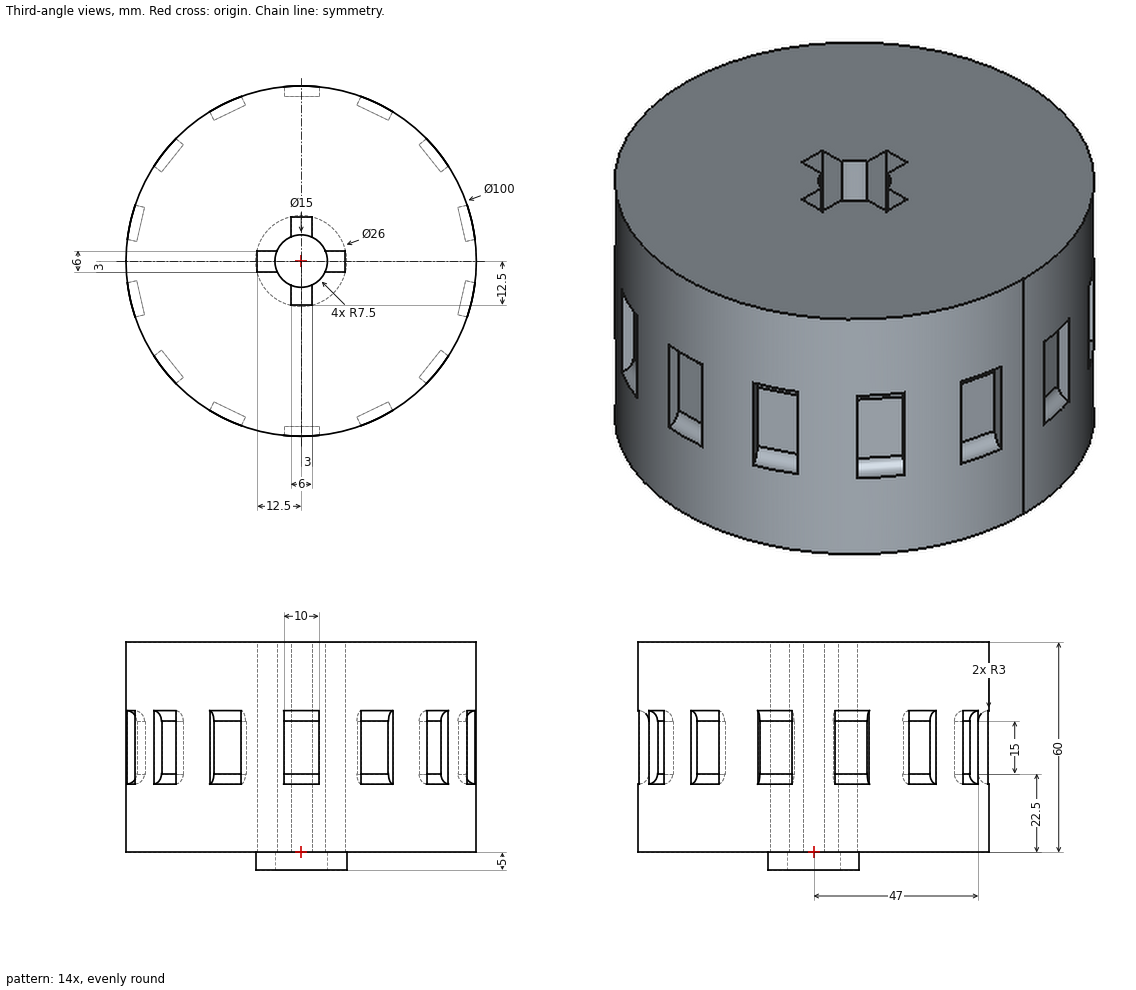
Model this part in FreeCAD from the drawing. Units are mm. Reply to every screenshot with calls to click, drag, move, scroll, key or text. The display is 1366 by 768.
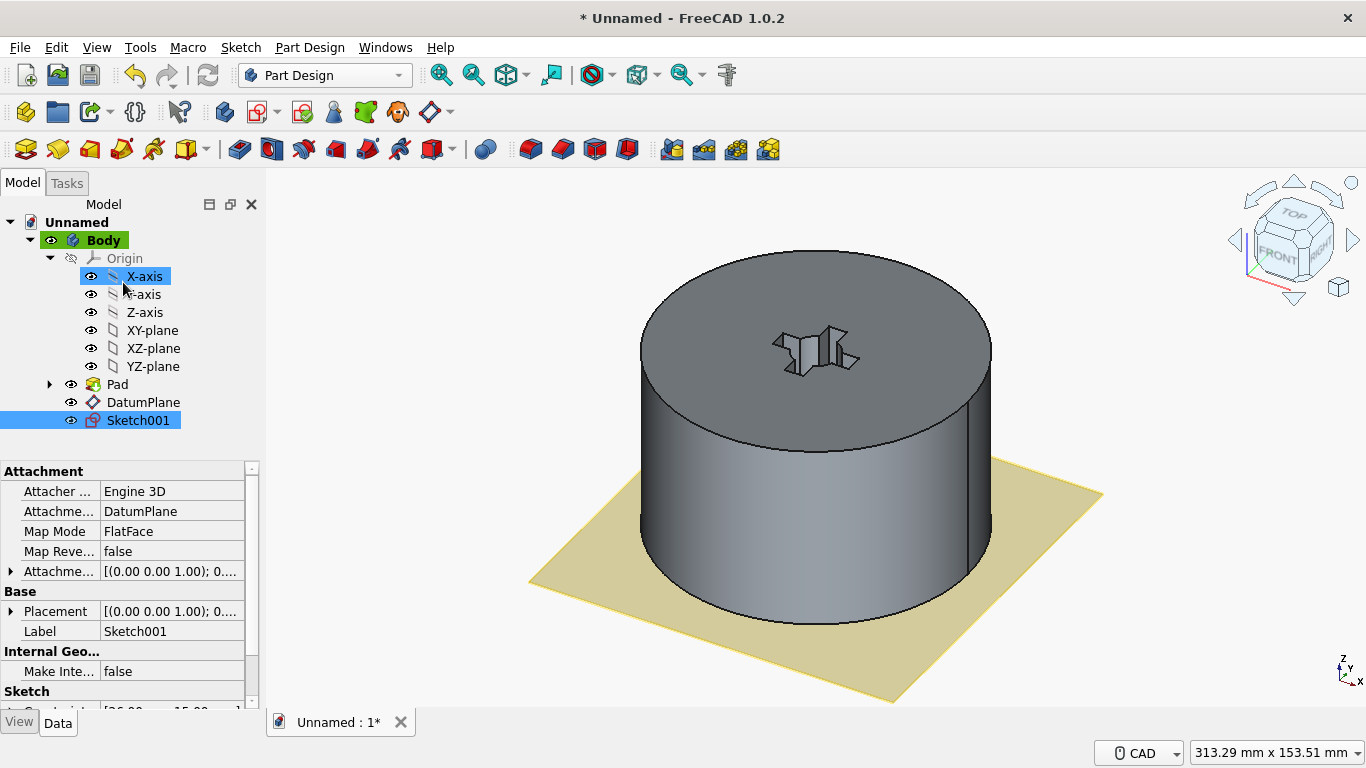
click(26, 150)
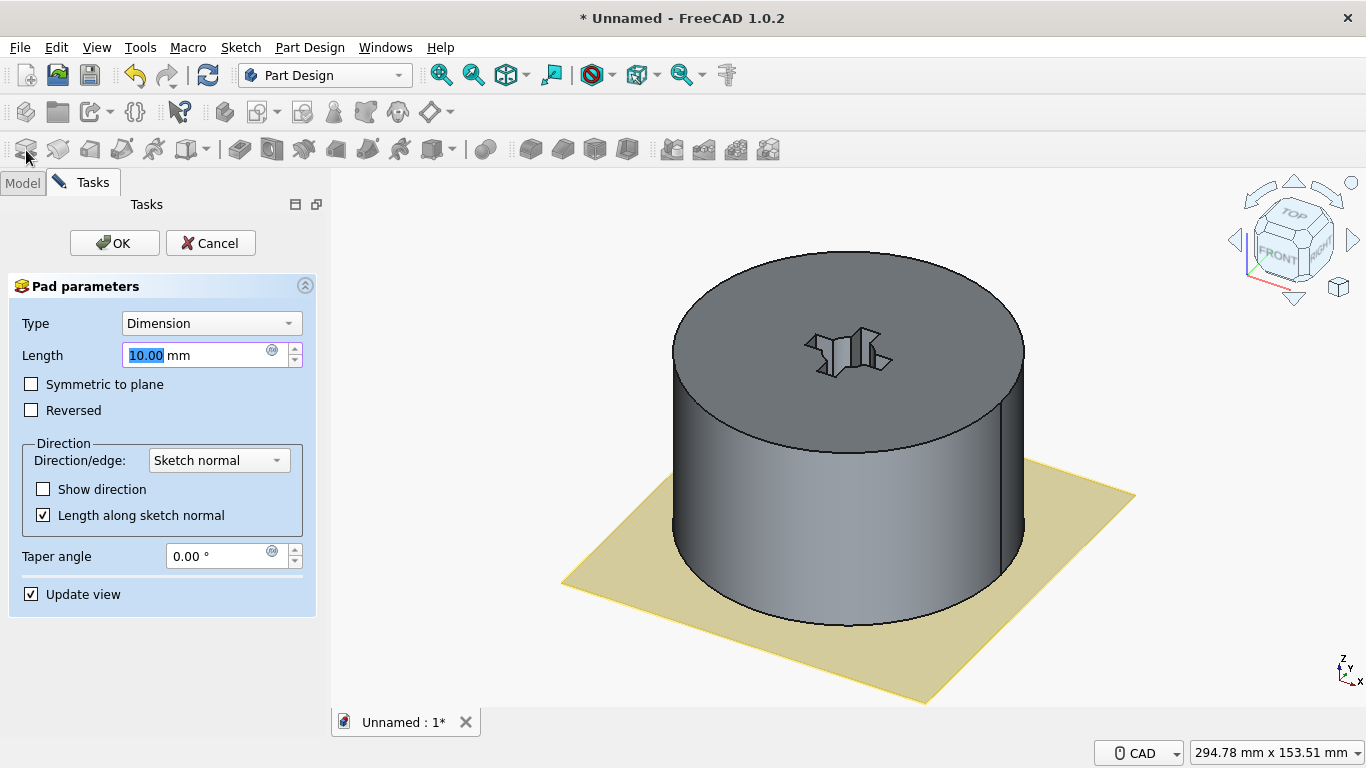
text(5)
key(Tab)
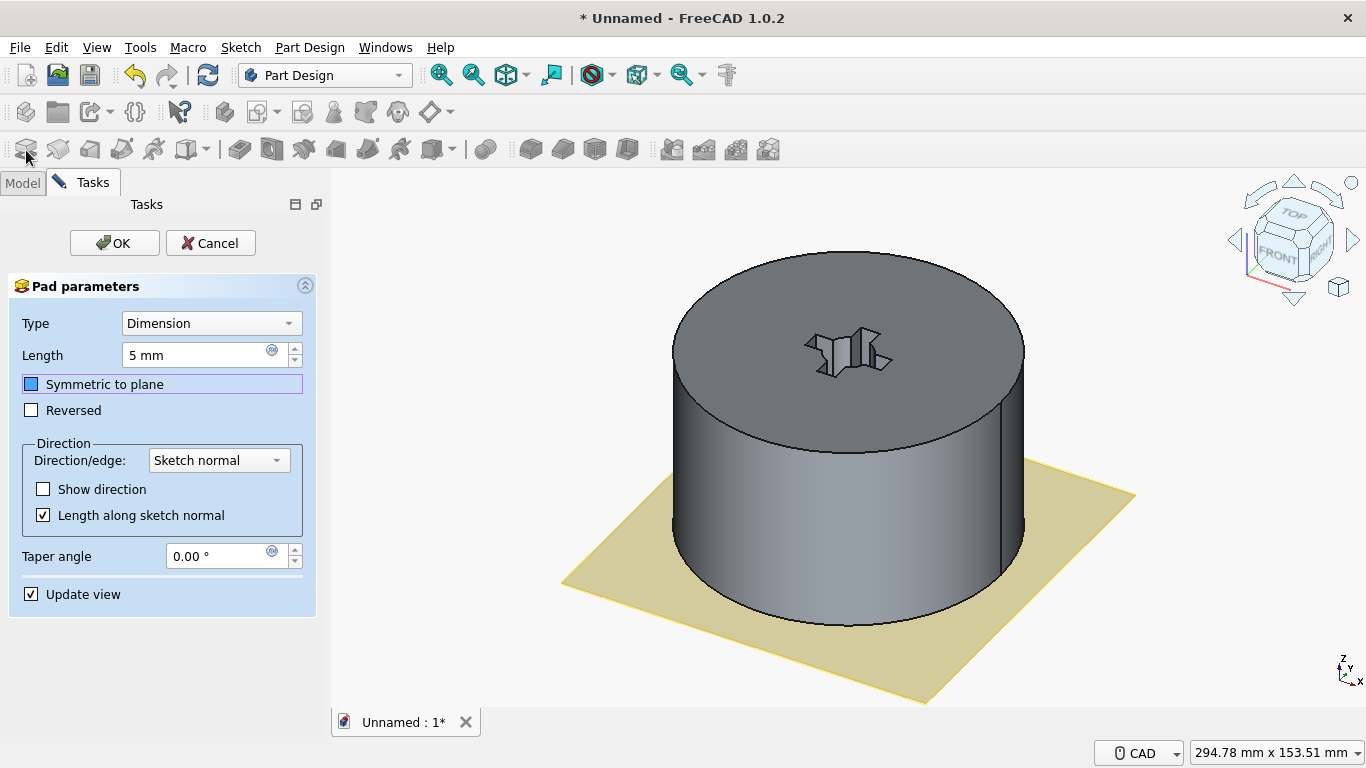
click(115, 243)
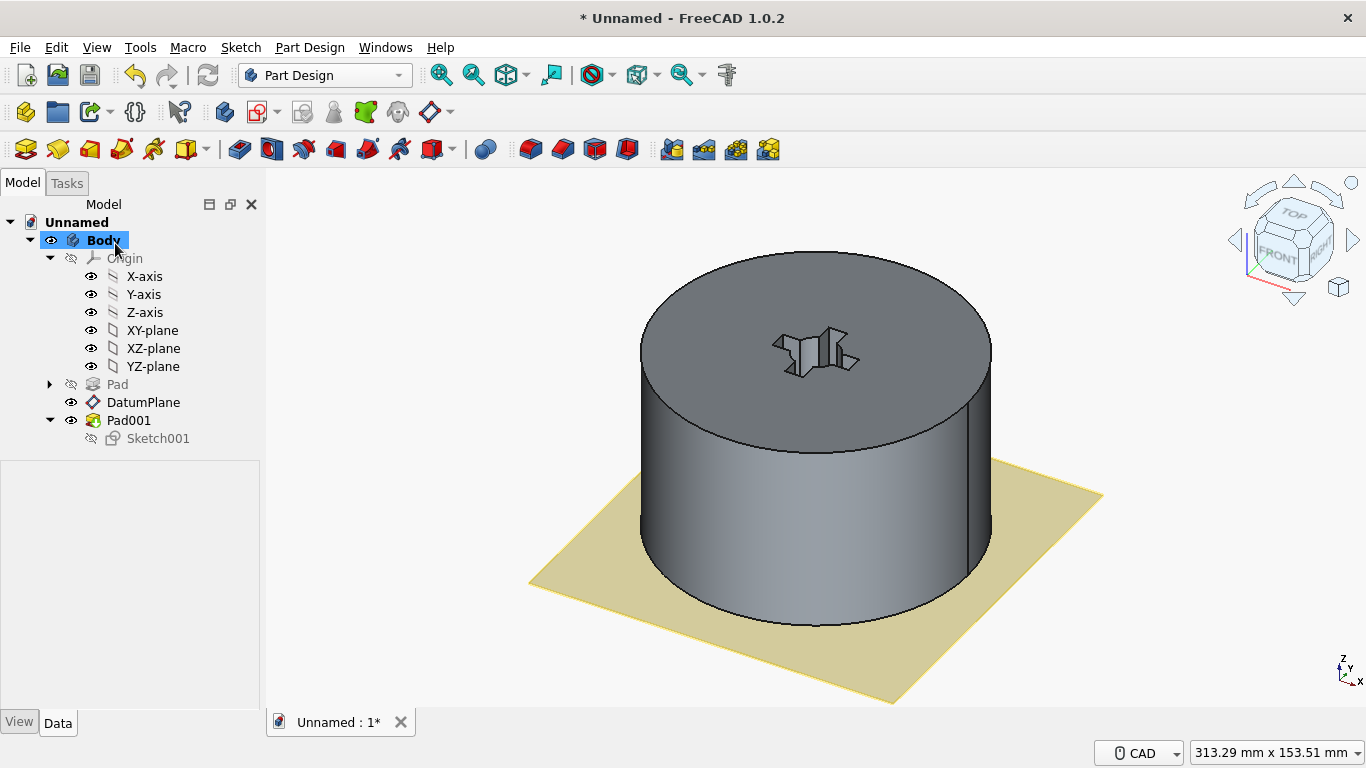
click(116, 402)
key(space)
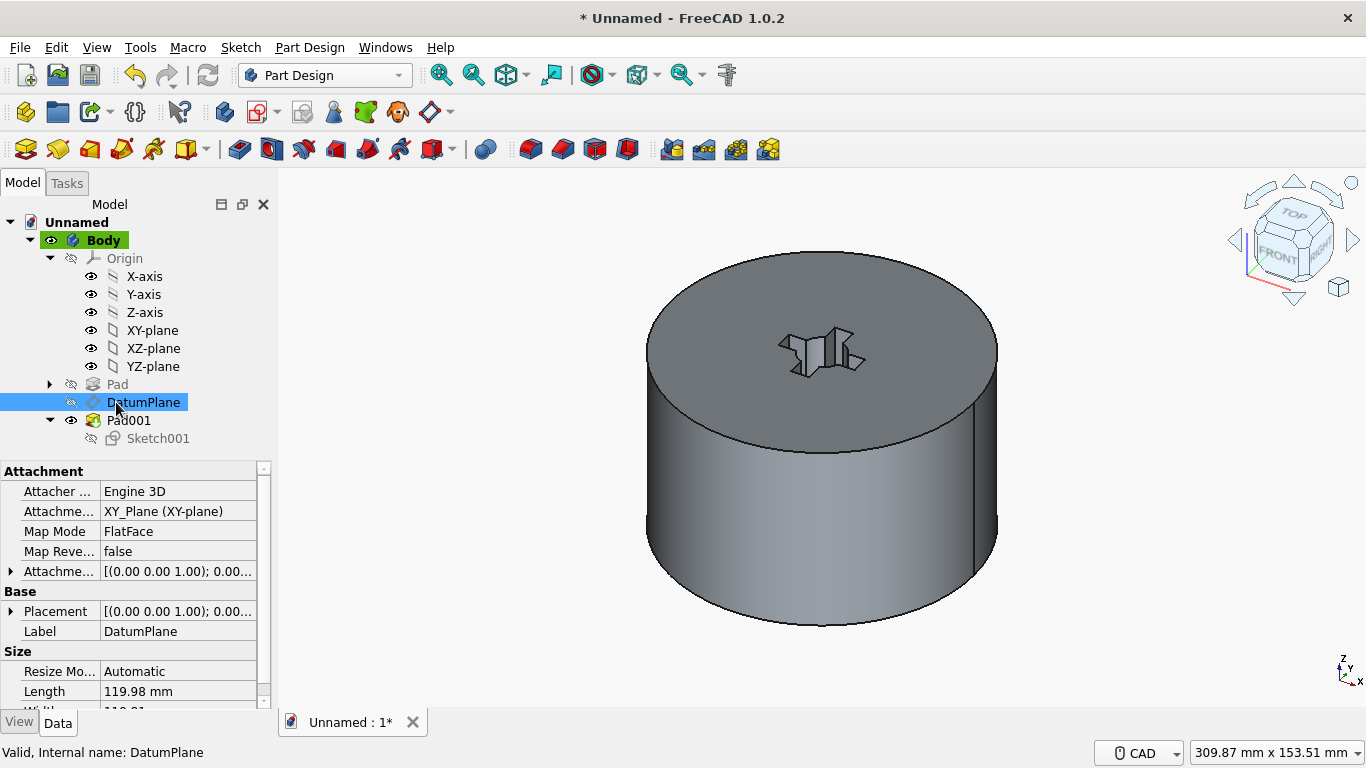
click(318, 667)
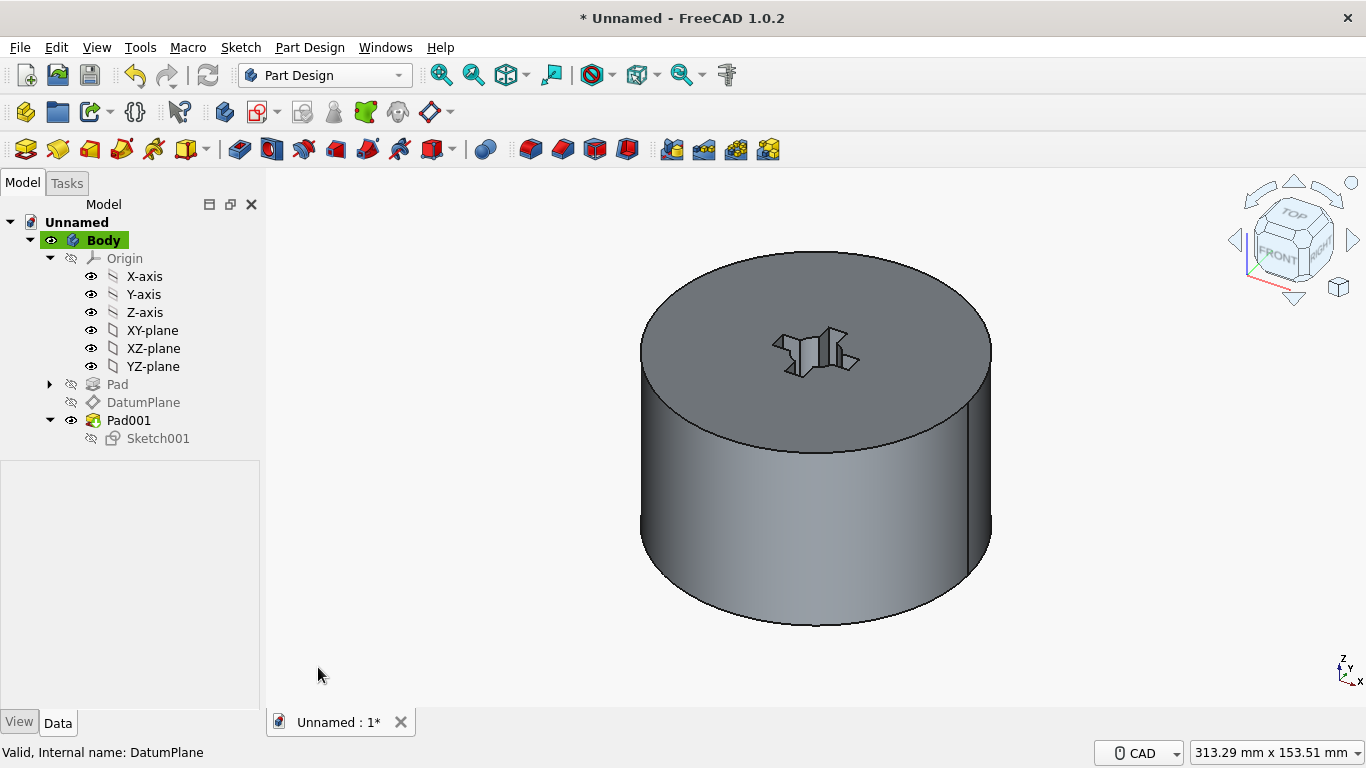
click(258, 112)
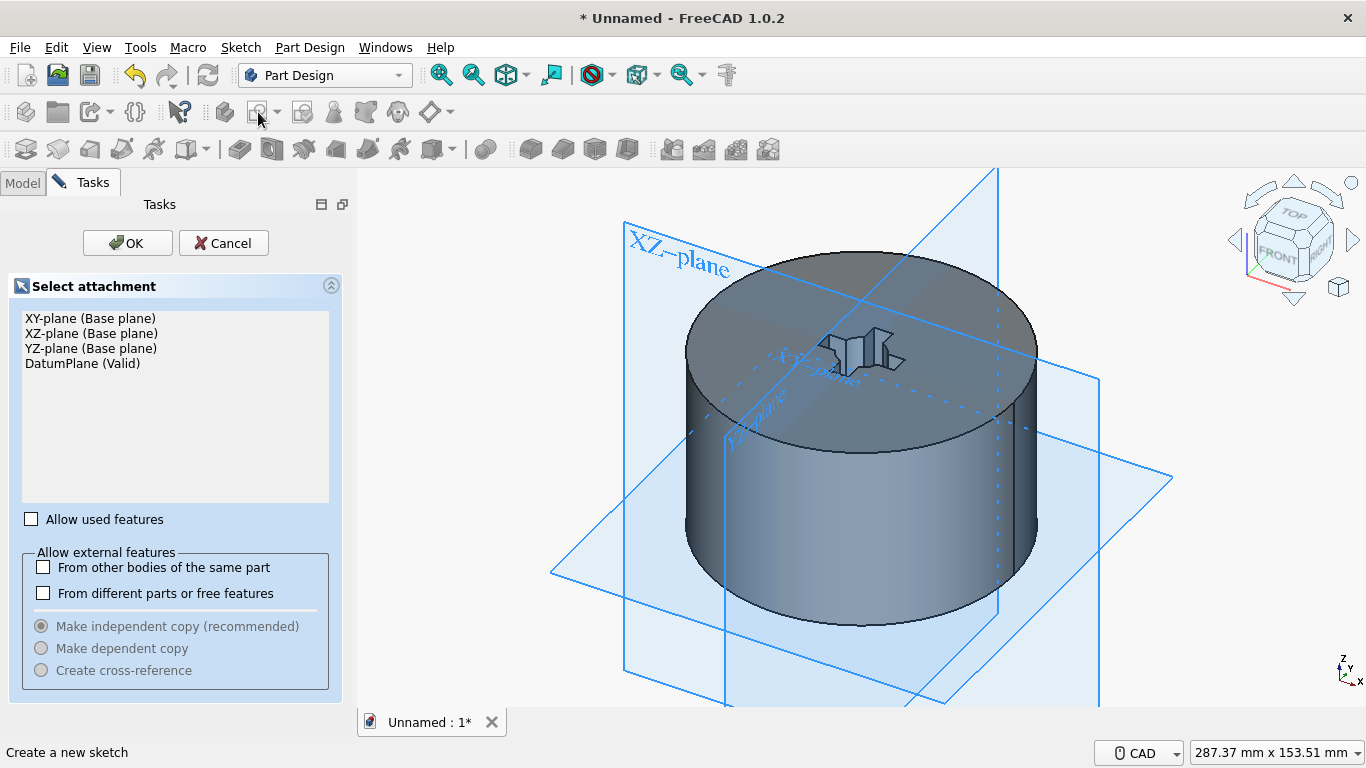
click(82, 348)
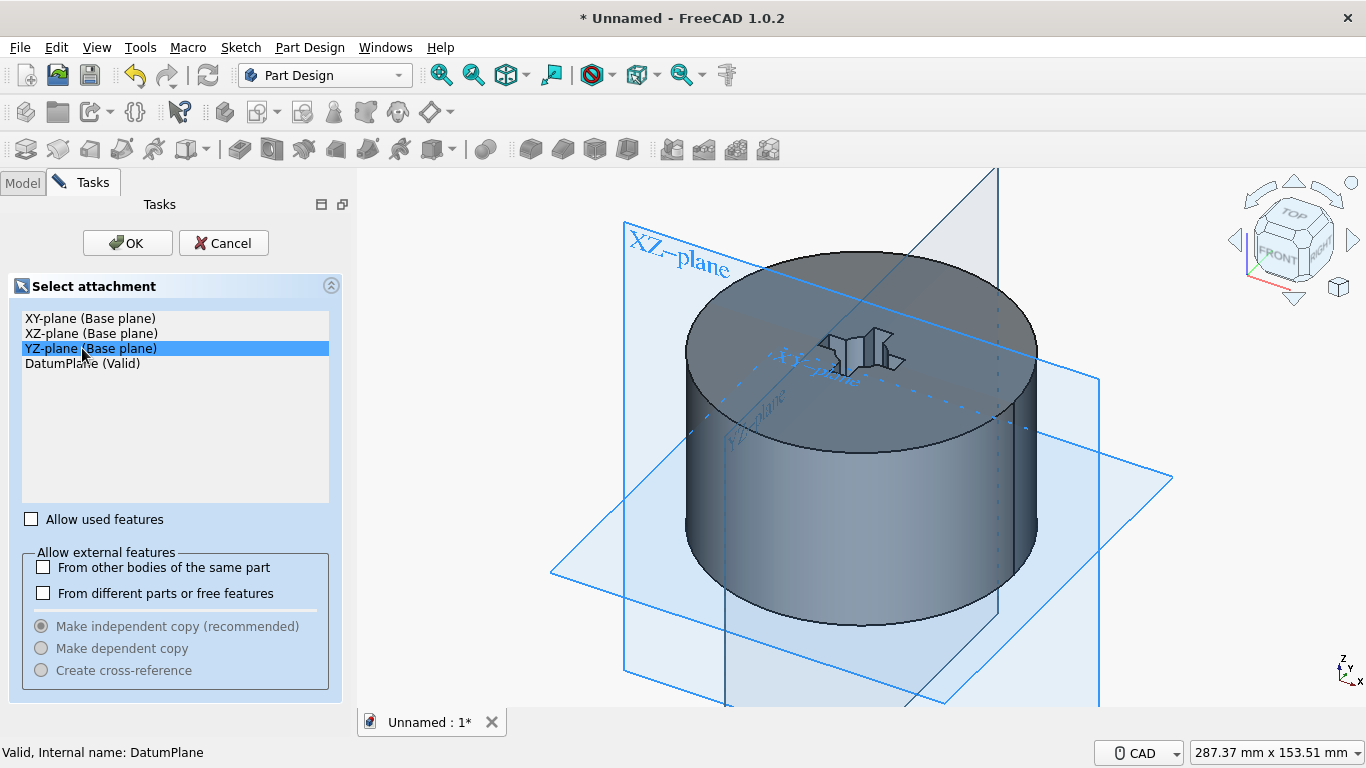
click(128, 243)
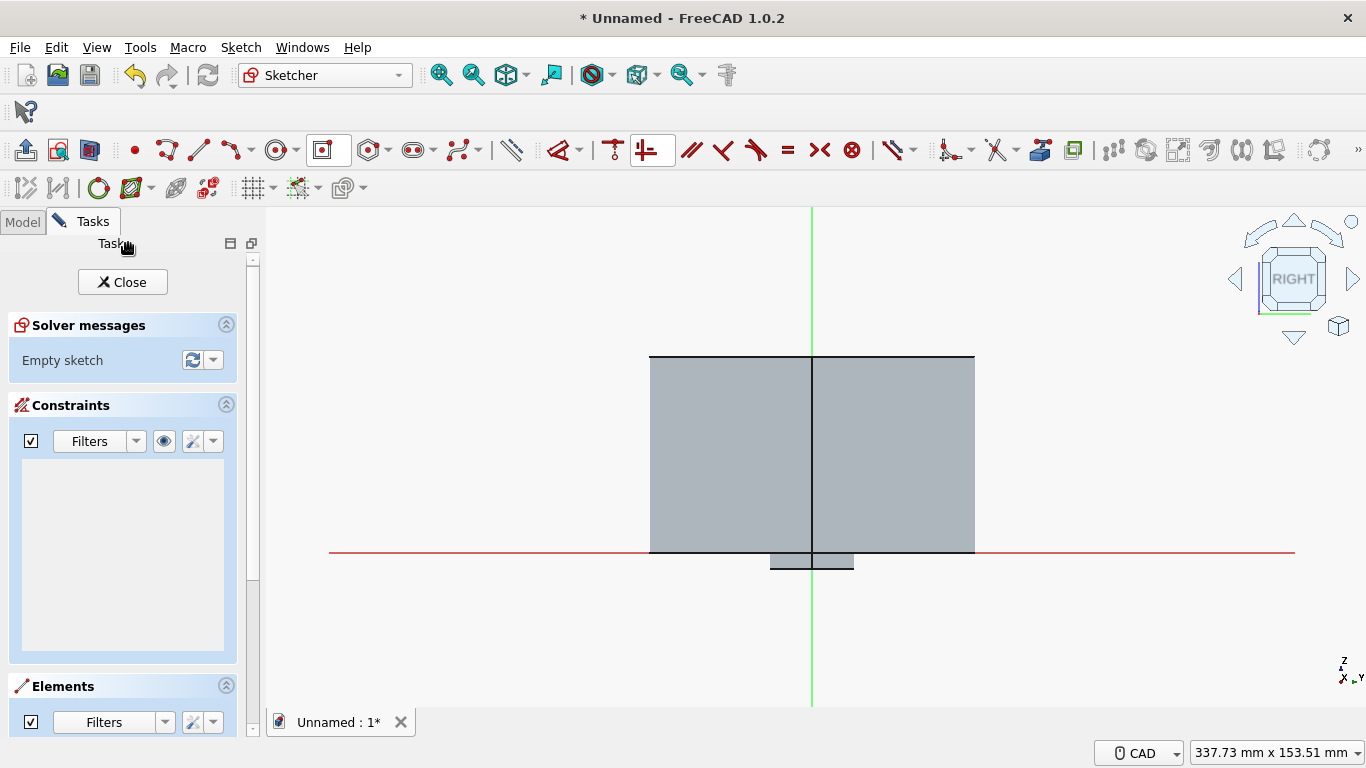
click(90, 150)